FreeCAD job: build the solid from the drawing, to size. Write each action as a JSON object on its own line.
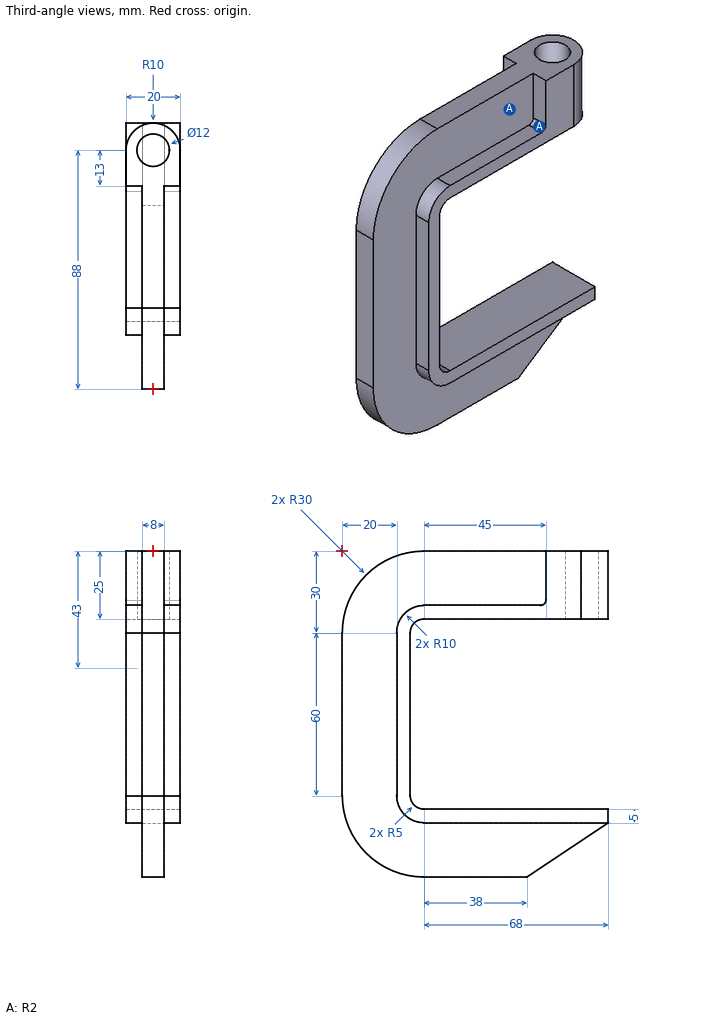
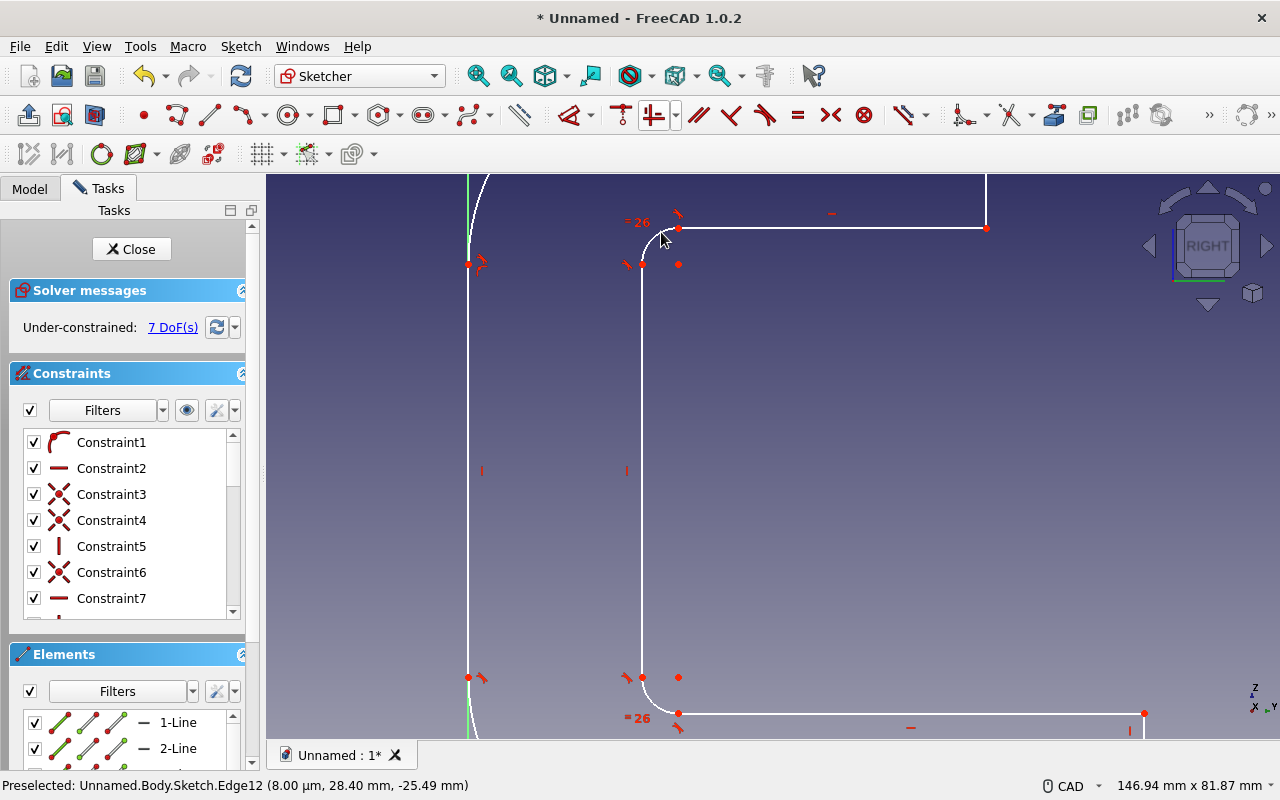
{"action": "key", "text": "d"}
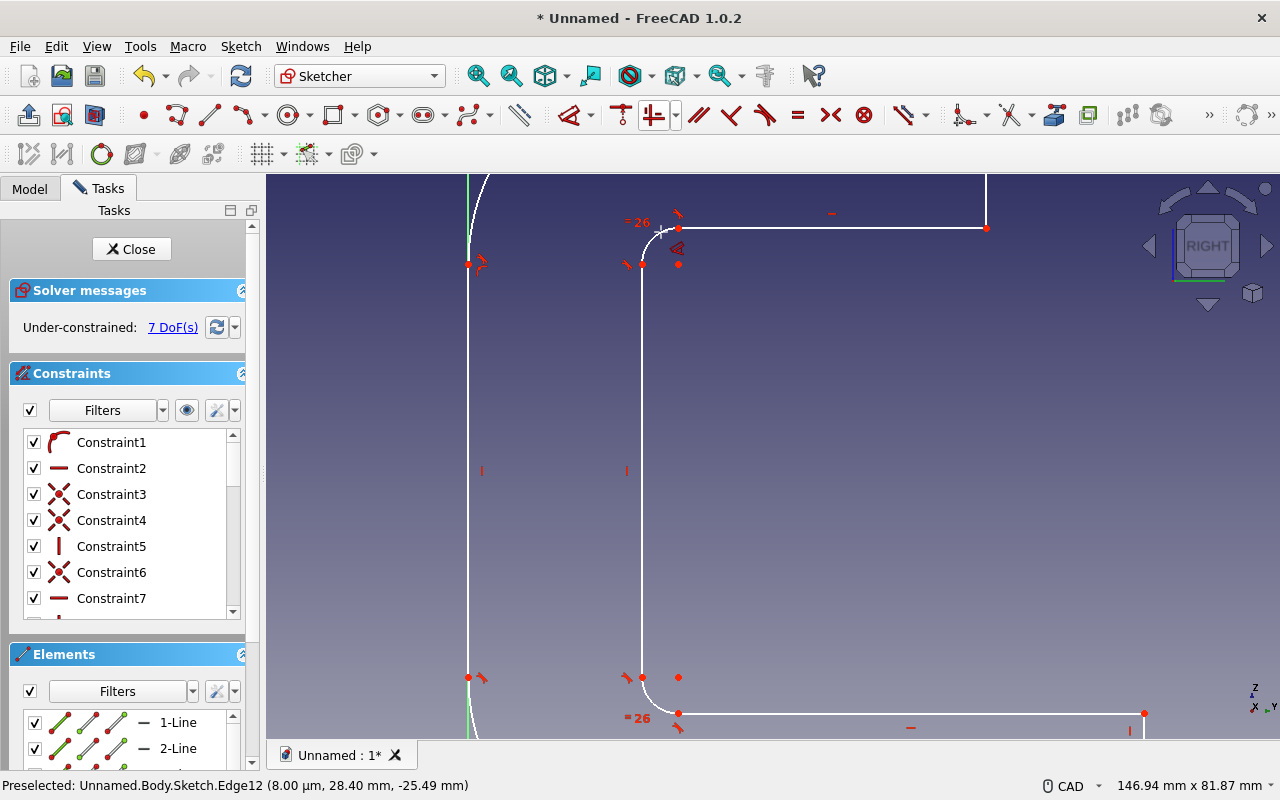
{"action": "scroll", "coordinate": [621, 447], "scroll_direction": "down", "scroll_amount": 4}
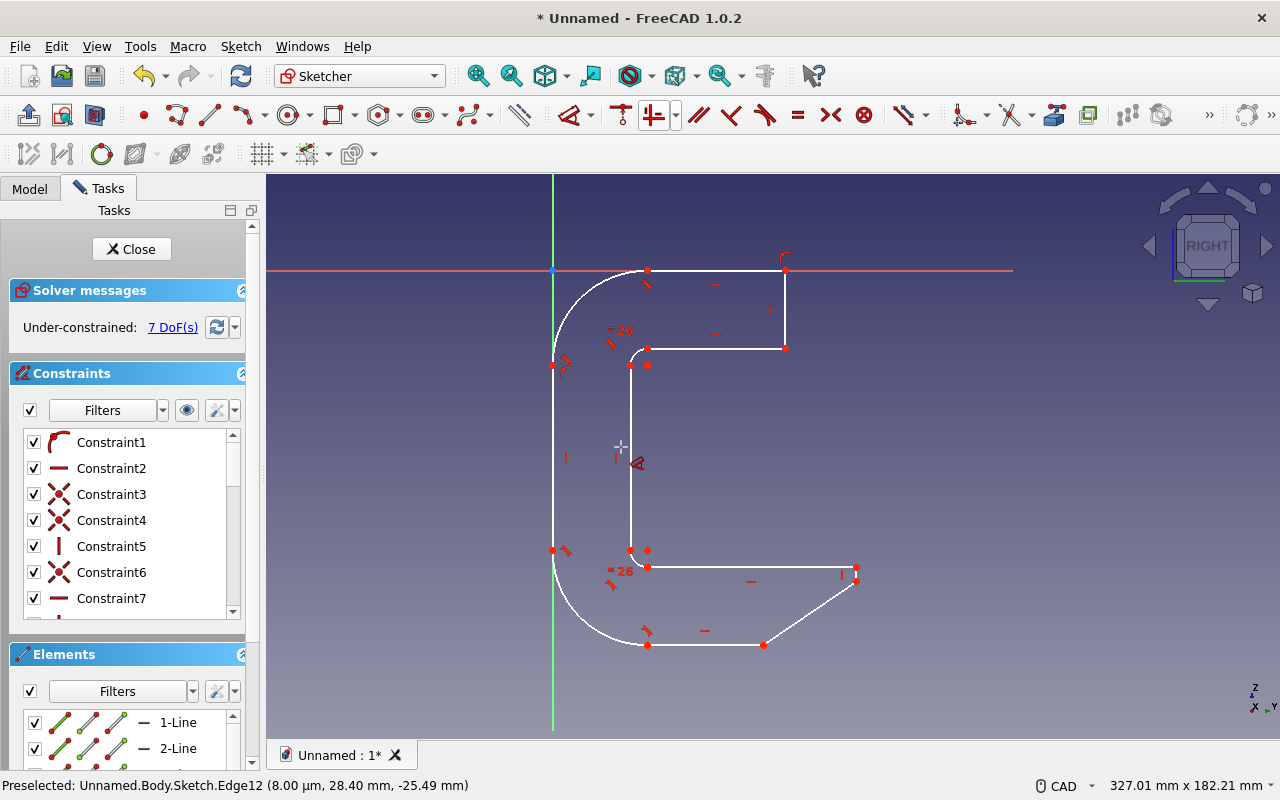
{"action": "scroll", "coordinate": [563, 594], "scroll_direction": "up", "scroll_amount": 2}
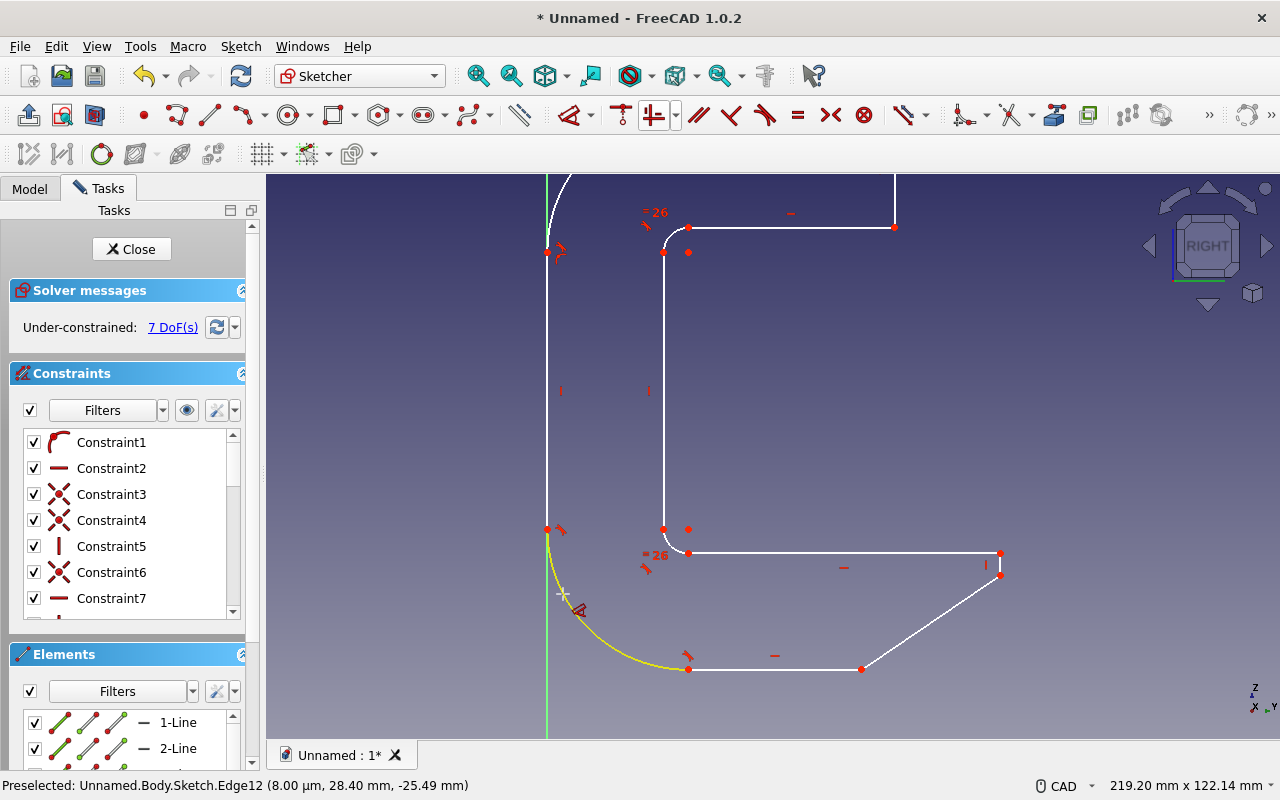
{"action": "left_click", "coordinate": [563, 593]}
{"action": "left_click", "coordinate": [516, 524]}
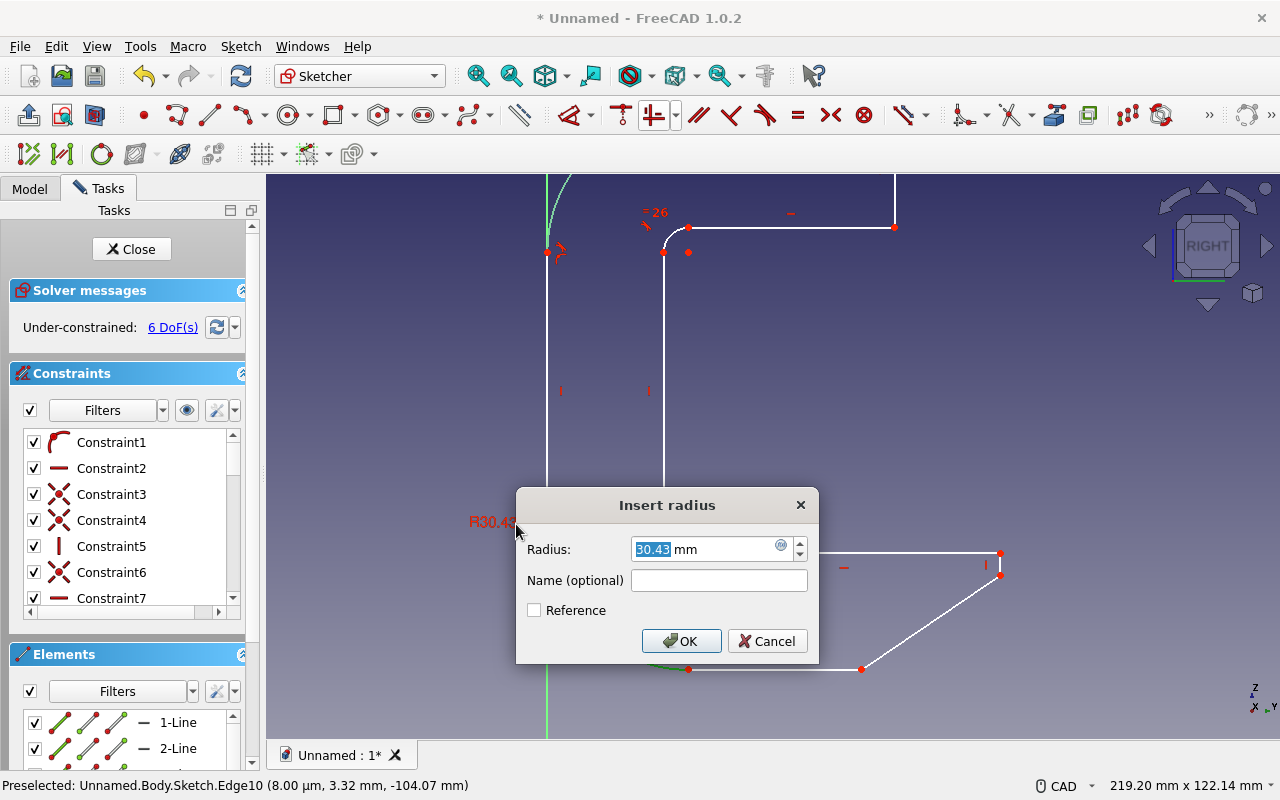
{"action": "type", "text": "30"}
{"action": "key", "text": "Return"}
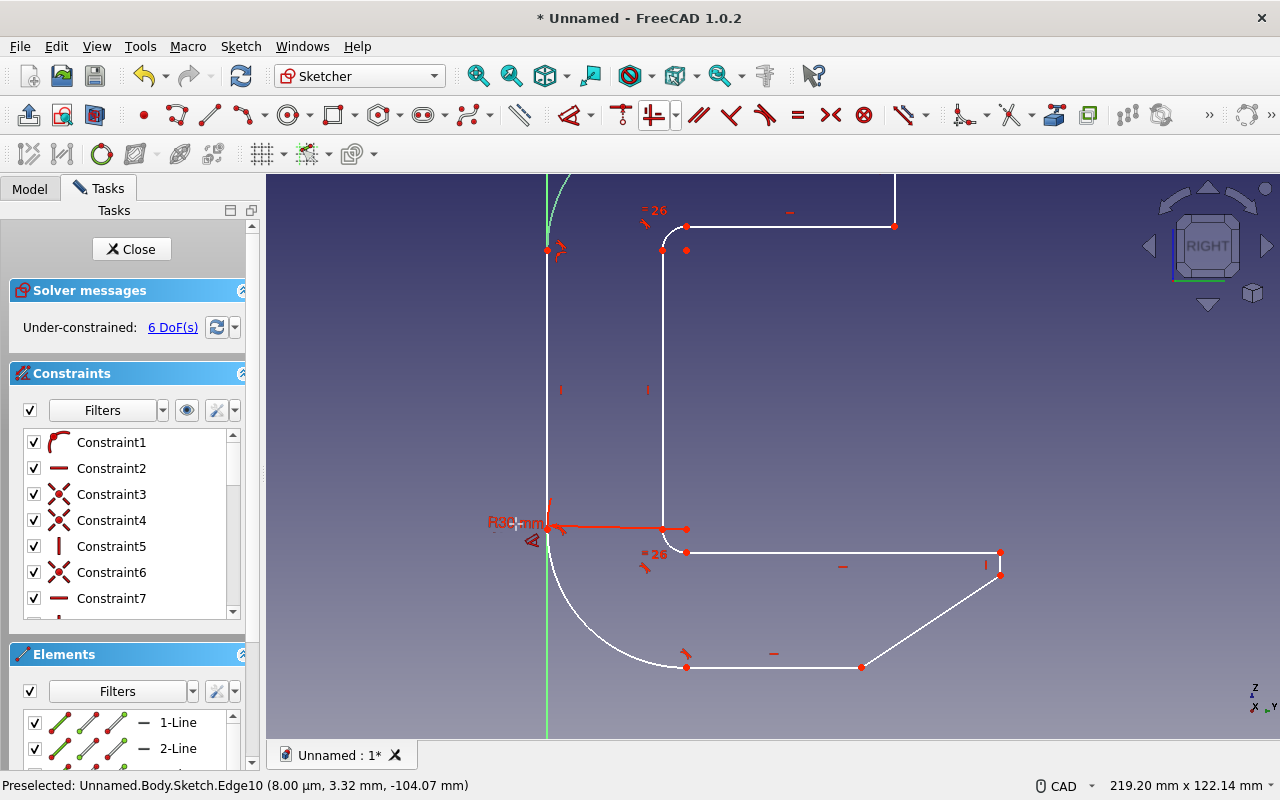
{"action": "scroll", "coordinate": [665, 540], "scroll_direction": "up", "scroll_amount": 3}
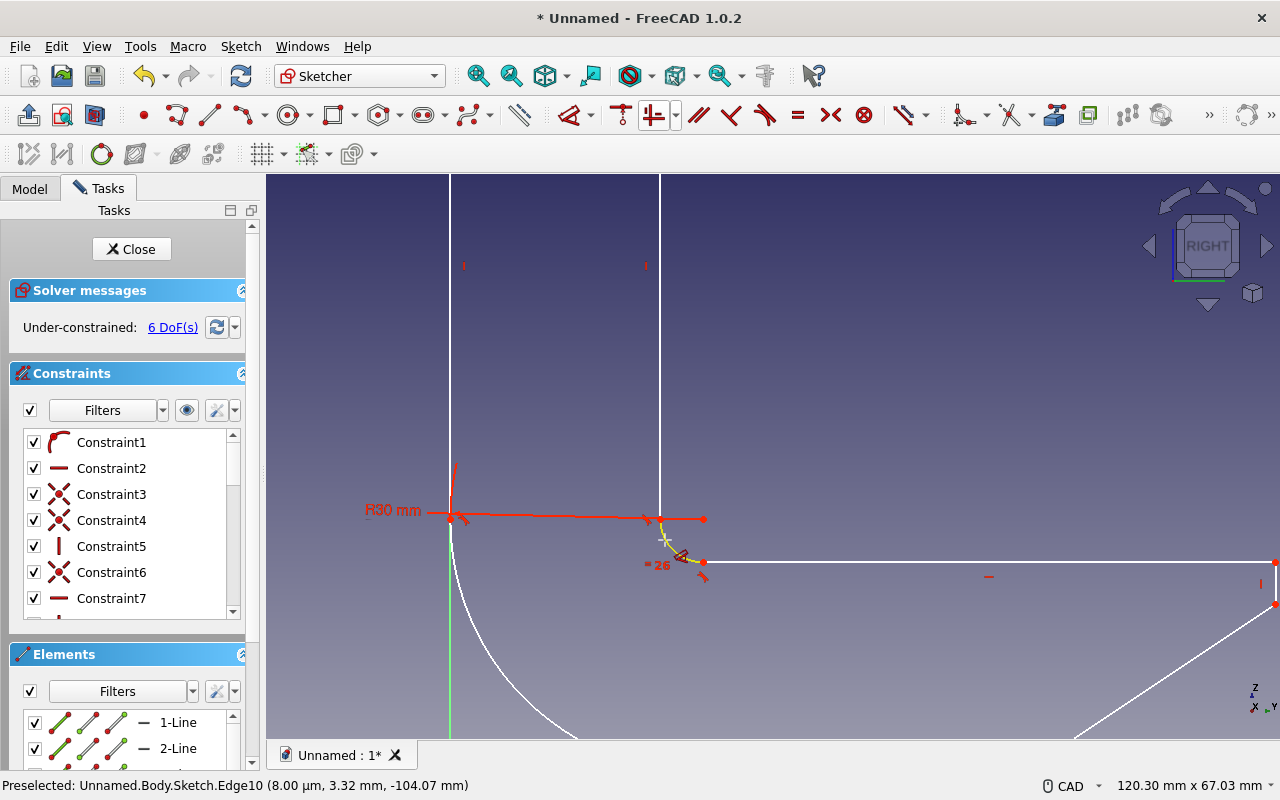
{"action": "left_click", "coordinate": [665, 539]}
{"action": "left_click", "coordinate": [636, 554]}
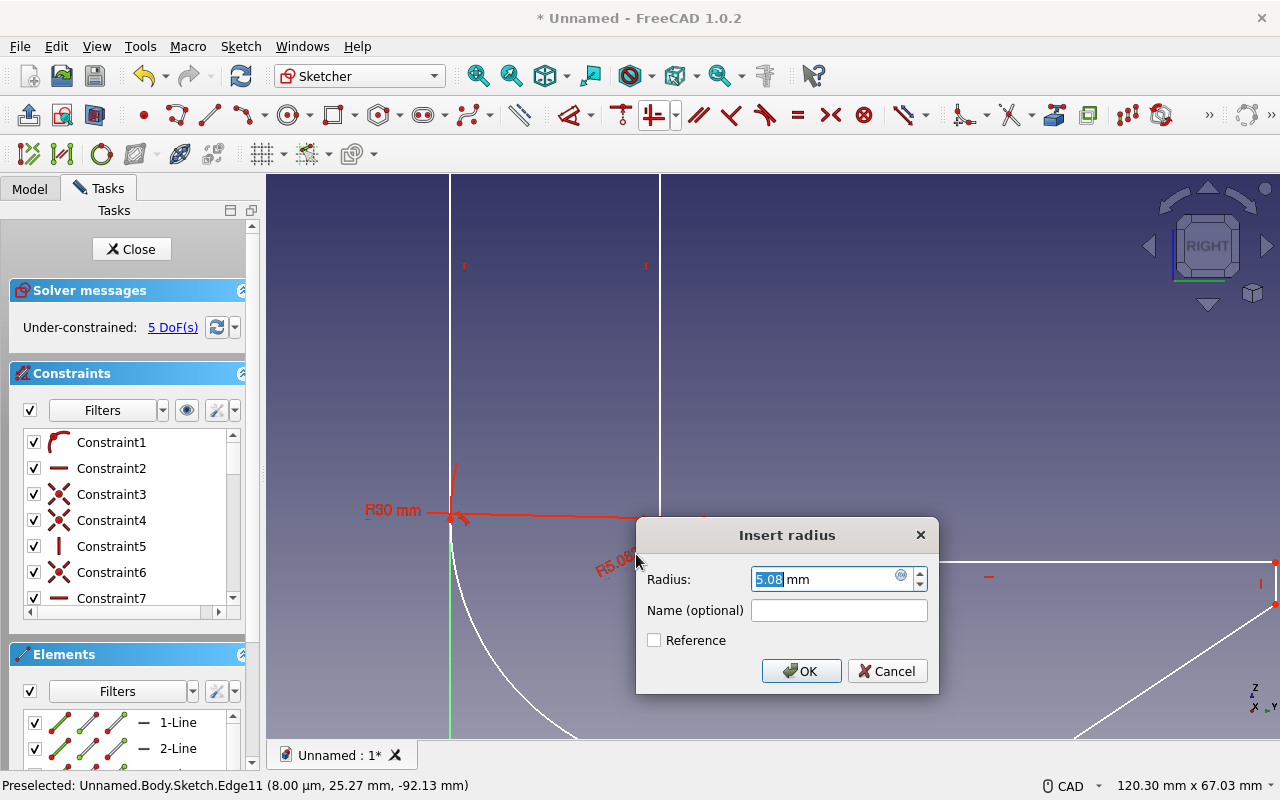
{"action": "type", "text": "5"}
{"action": "key", "text": "Return"}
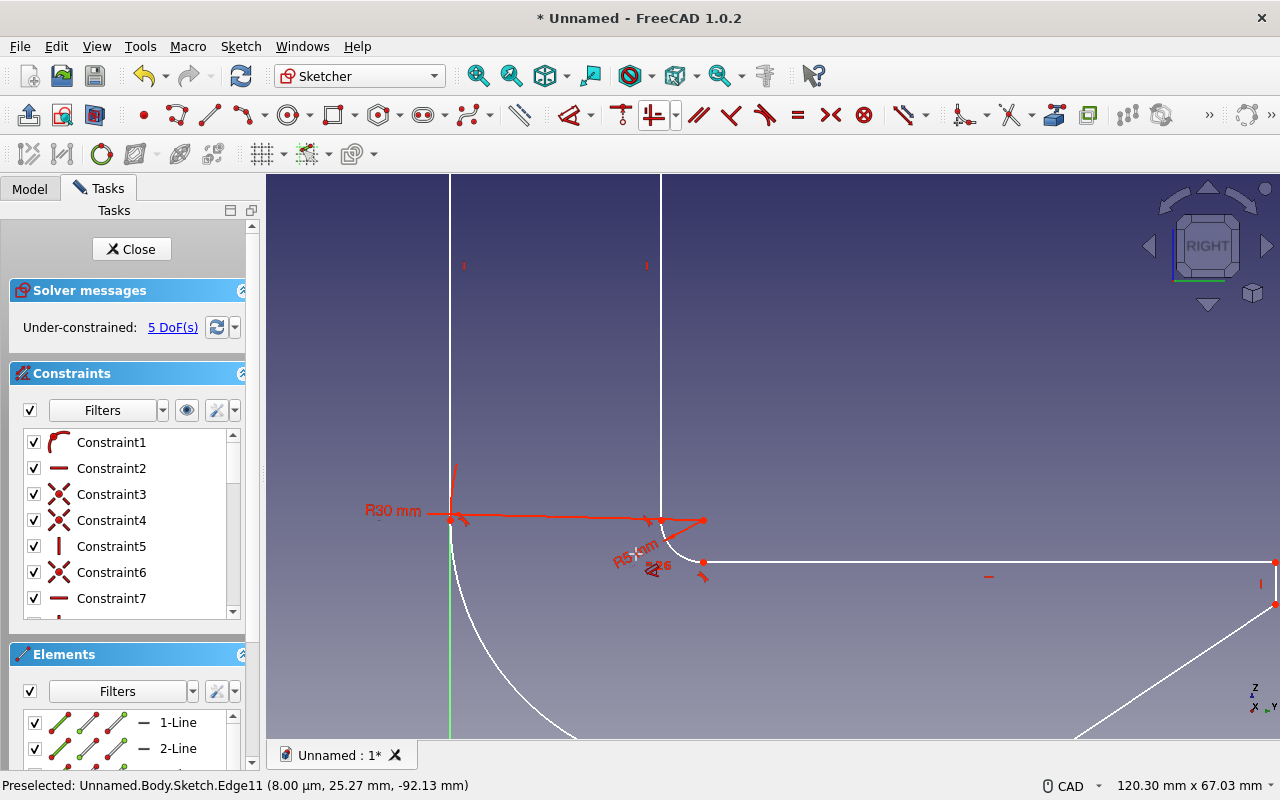
{"action": "scroll", "coordinate": [612, 568], "scroll_direction": "down", "scroll_amount": 5}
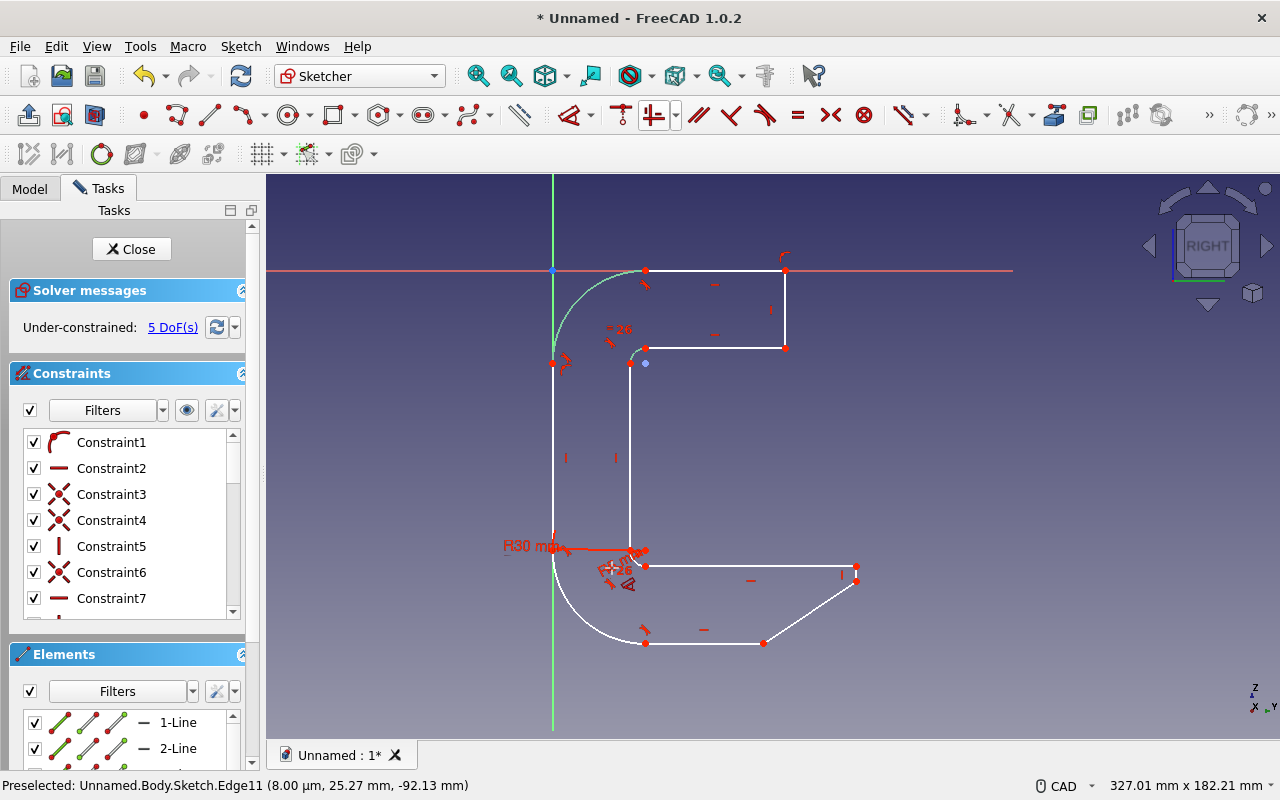
{"action": "scroll", "coordinate": [856, 577], "scroll_direction": "up", "scroll_amount": 6}